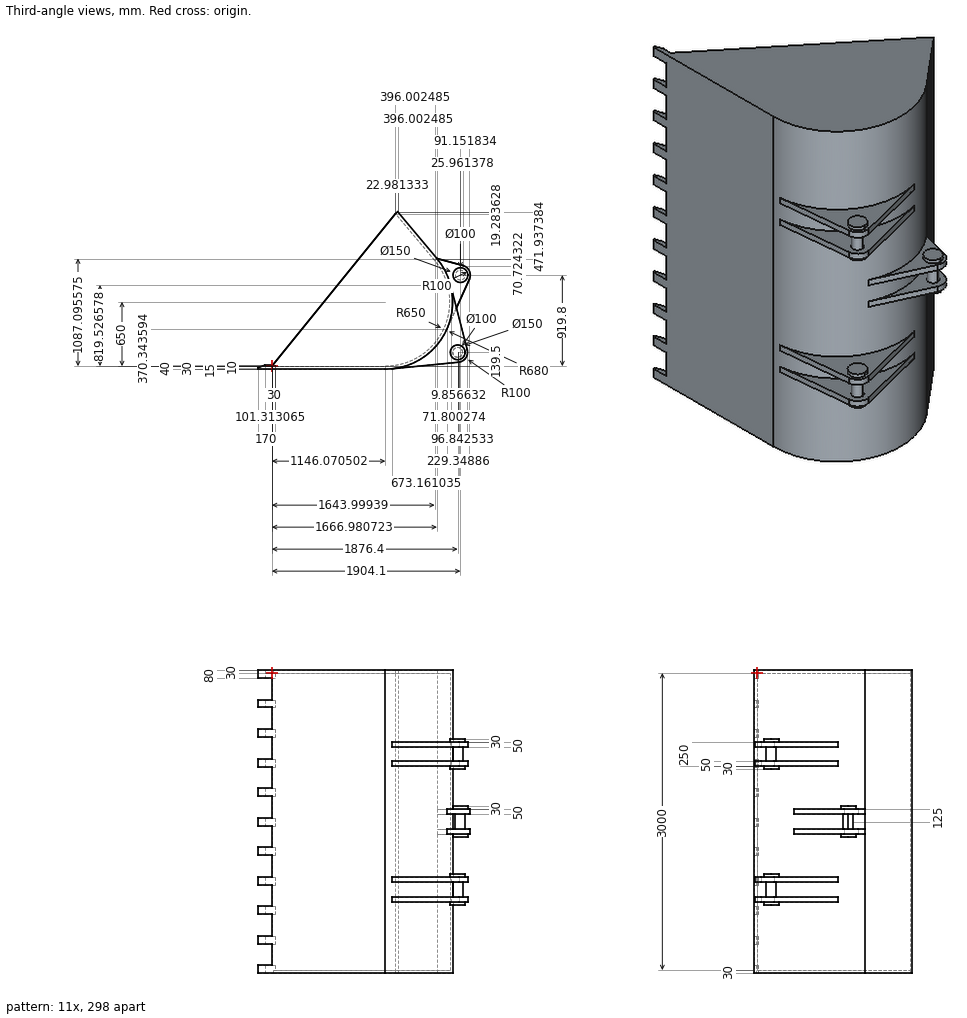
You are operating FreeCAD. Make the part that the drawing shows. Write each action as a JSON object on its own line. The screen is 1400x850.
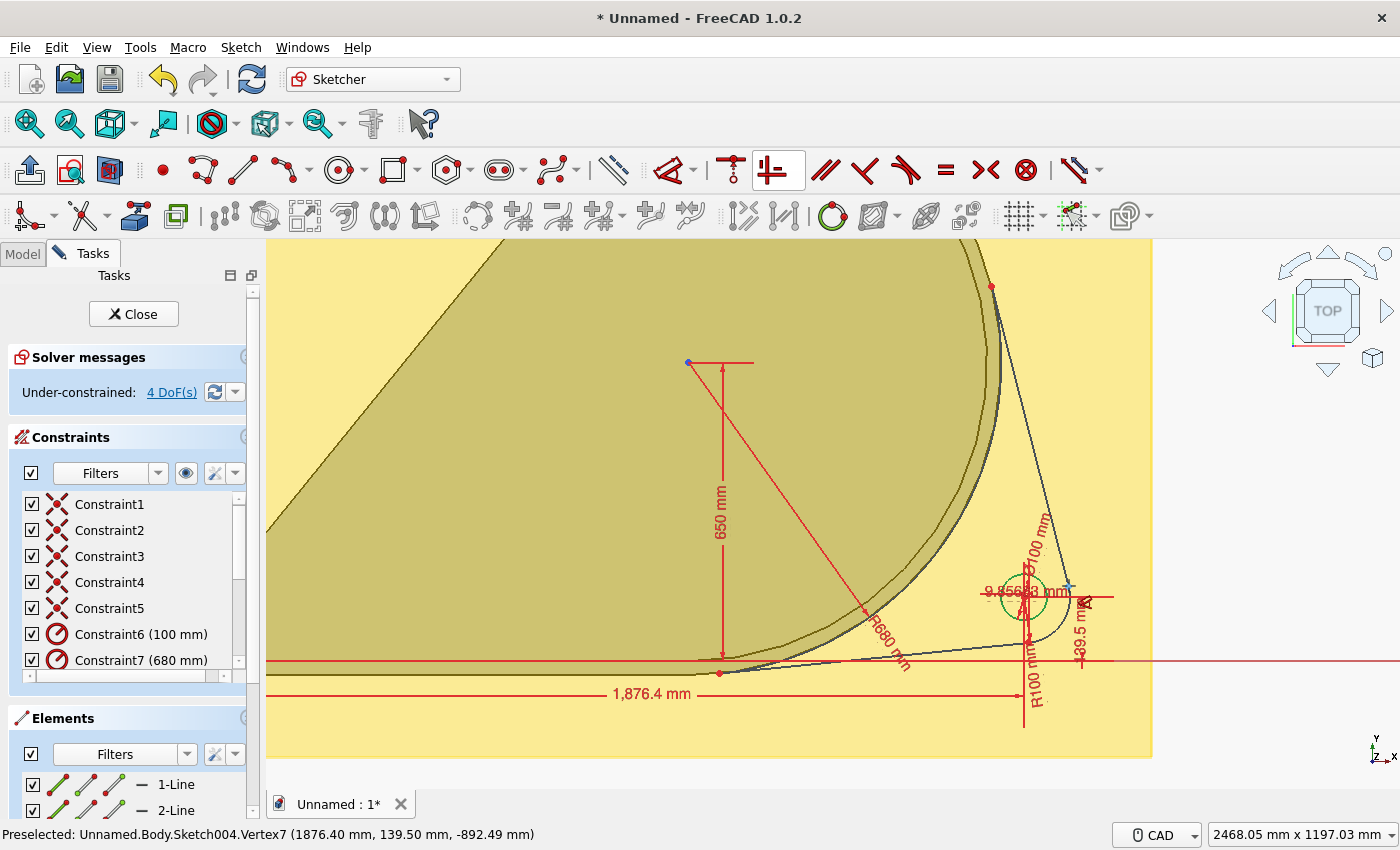
{"action": "left_click", "coordinate": [1069, 586]}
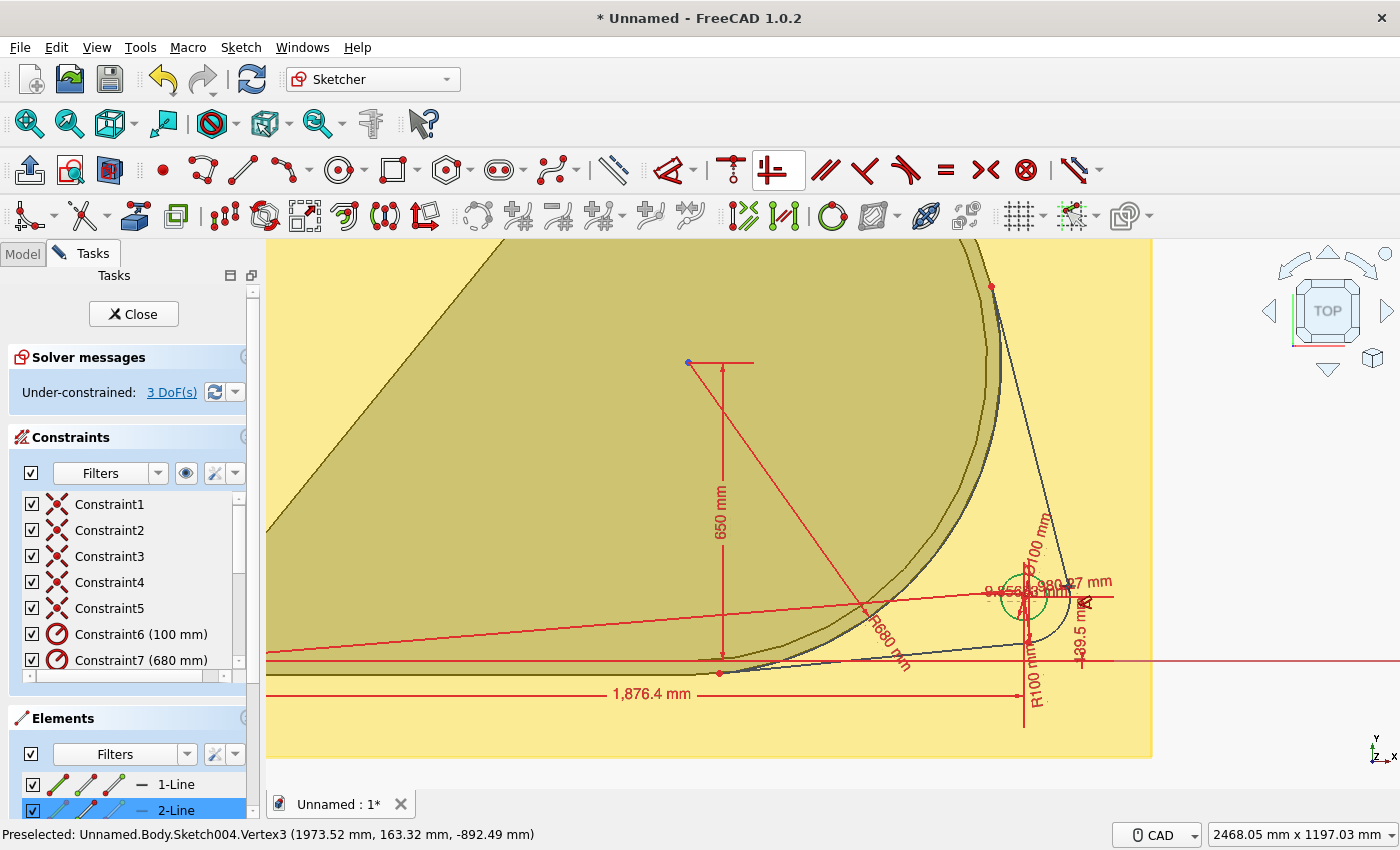
{"action": "left_click", "coordinate": [1024, 597]}
{"action": "left_click", "coordinate": [1031, 504]}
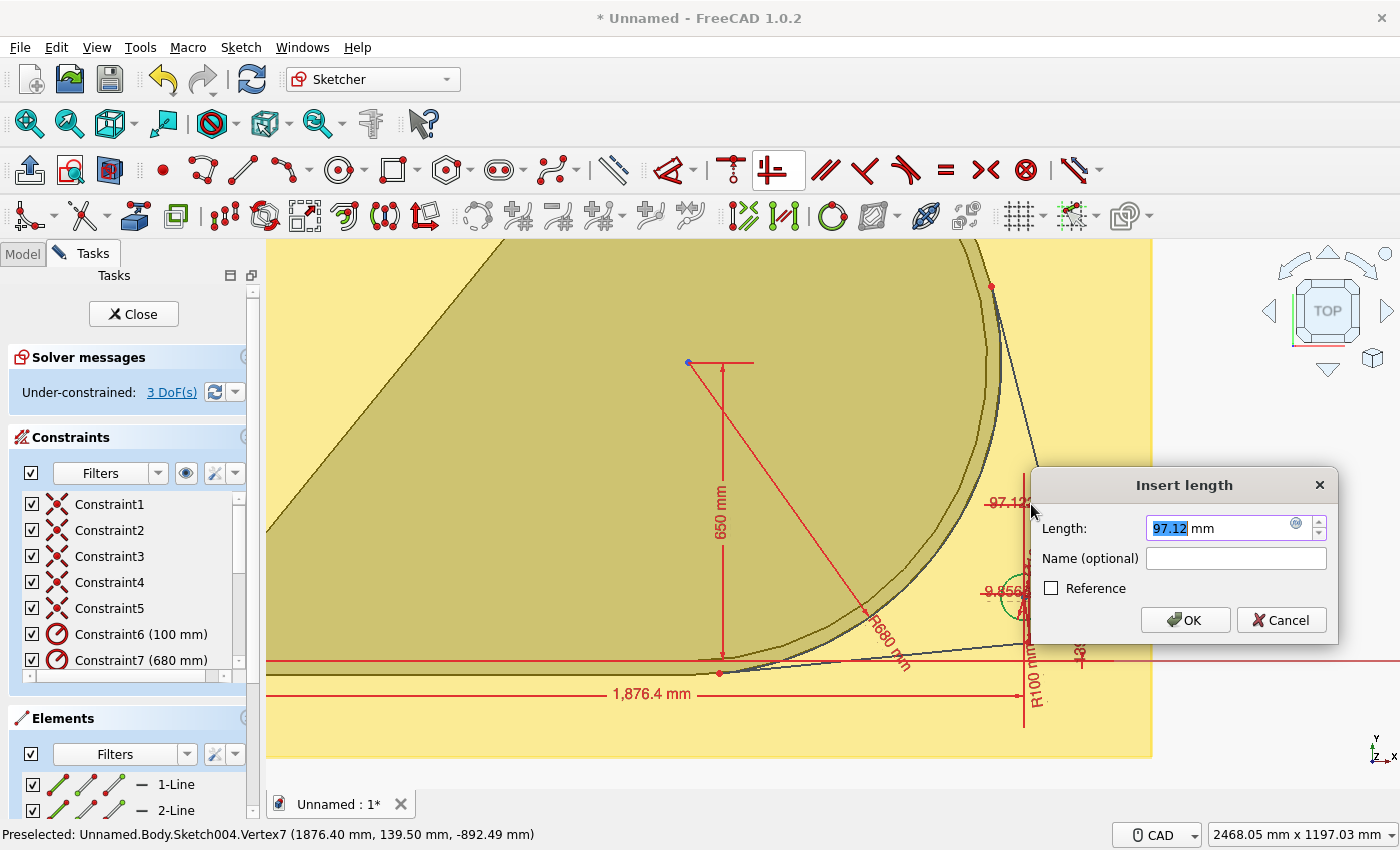
{"action": "type", "text": "96.842533"}
{"action": "key", "text": "Return"}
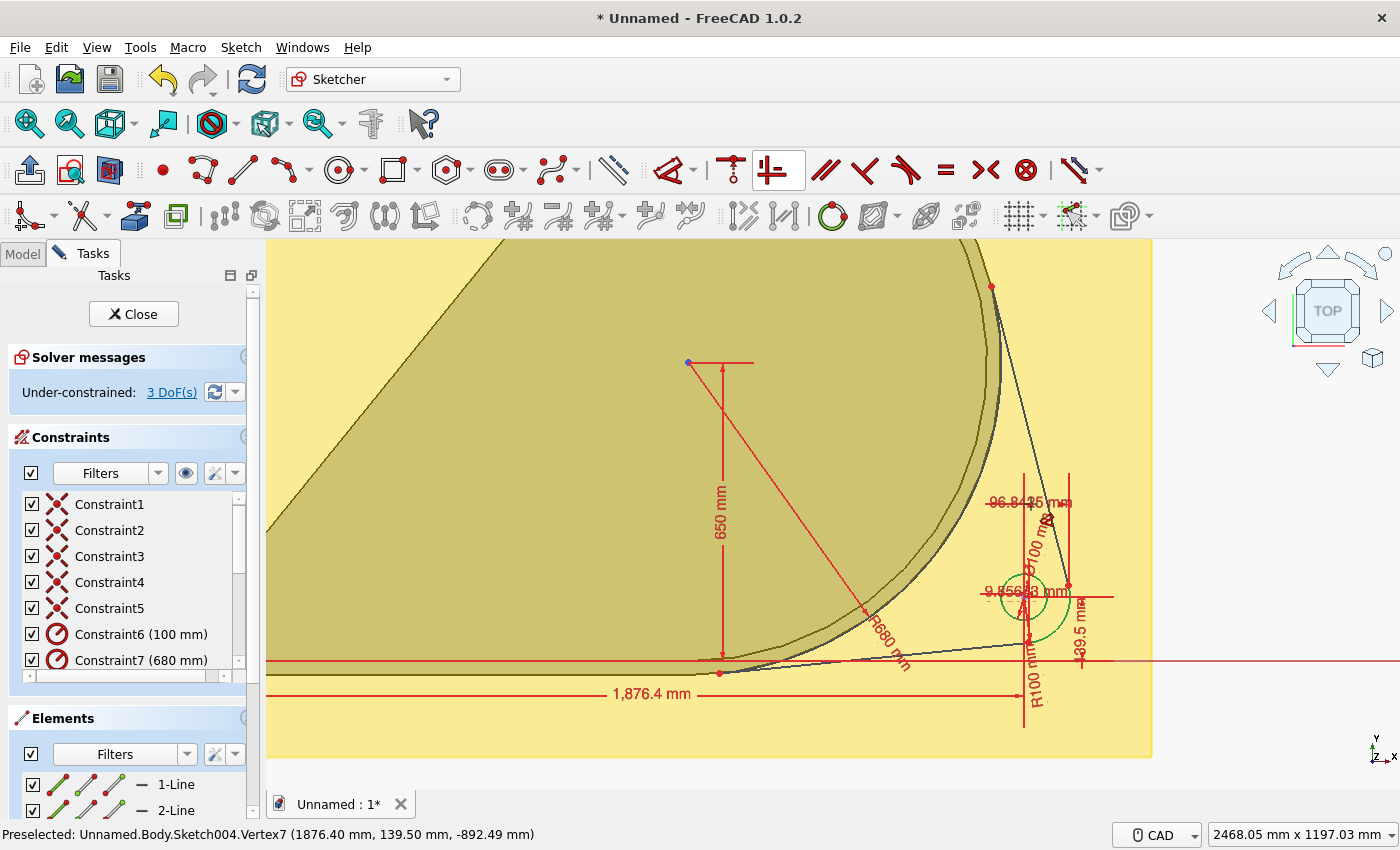
{"action": "left_click", "coordinate": [992, 286]}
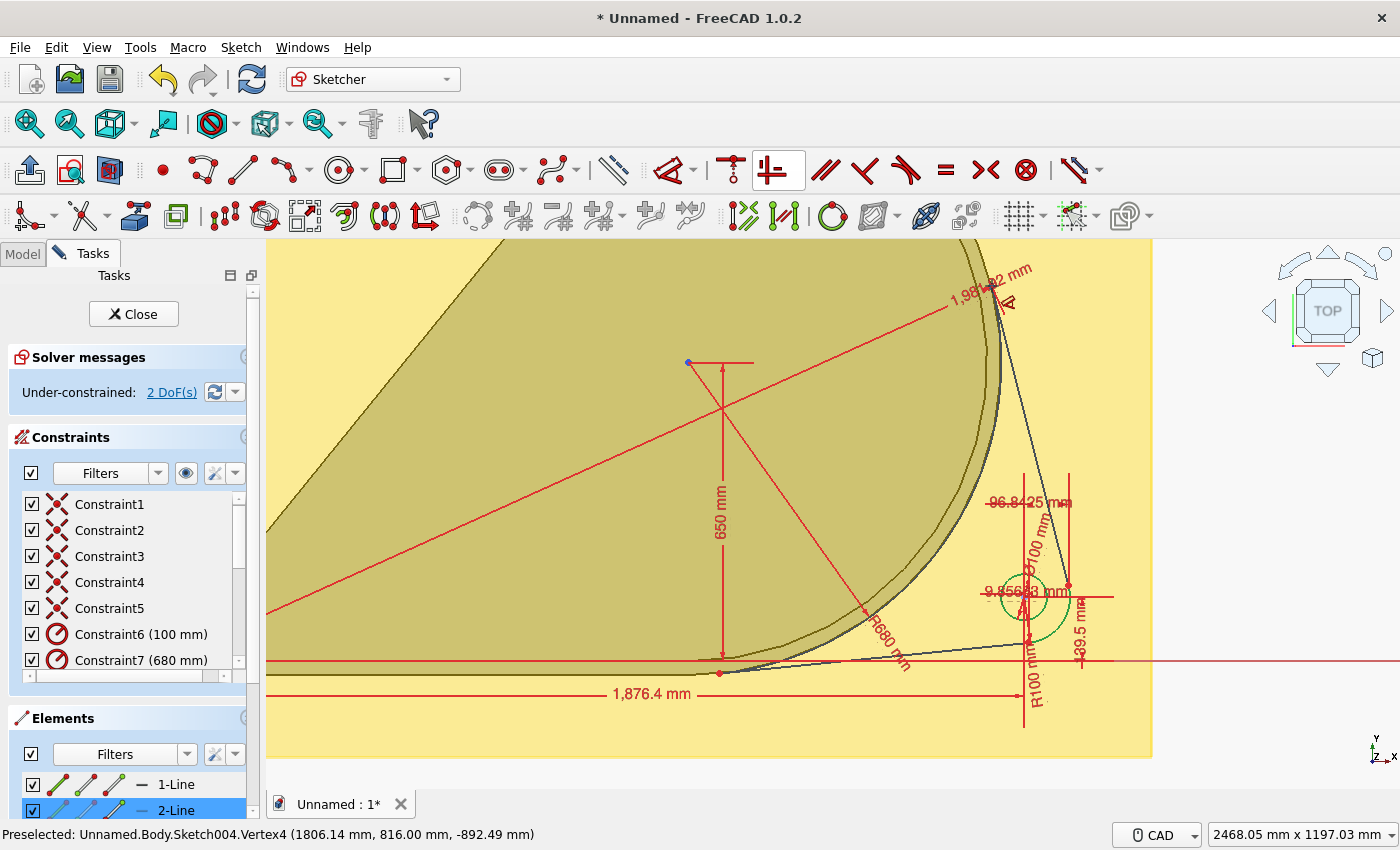
{"action": "left_click", "coordinate": [1024, 597]}
{"action": "left_click", "coordinate": [1008, 631]}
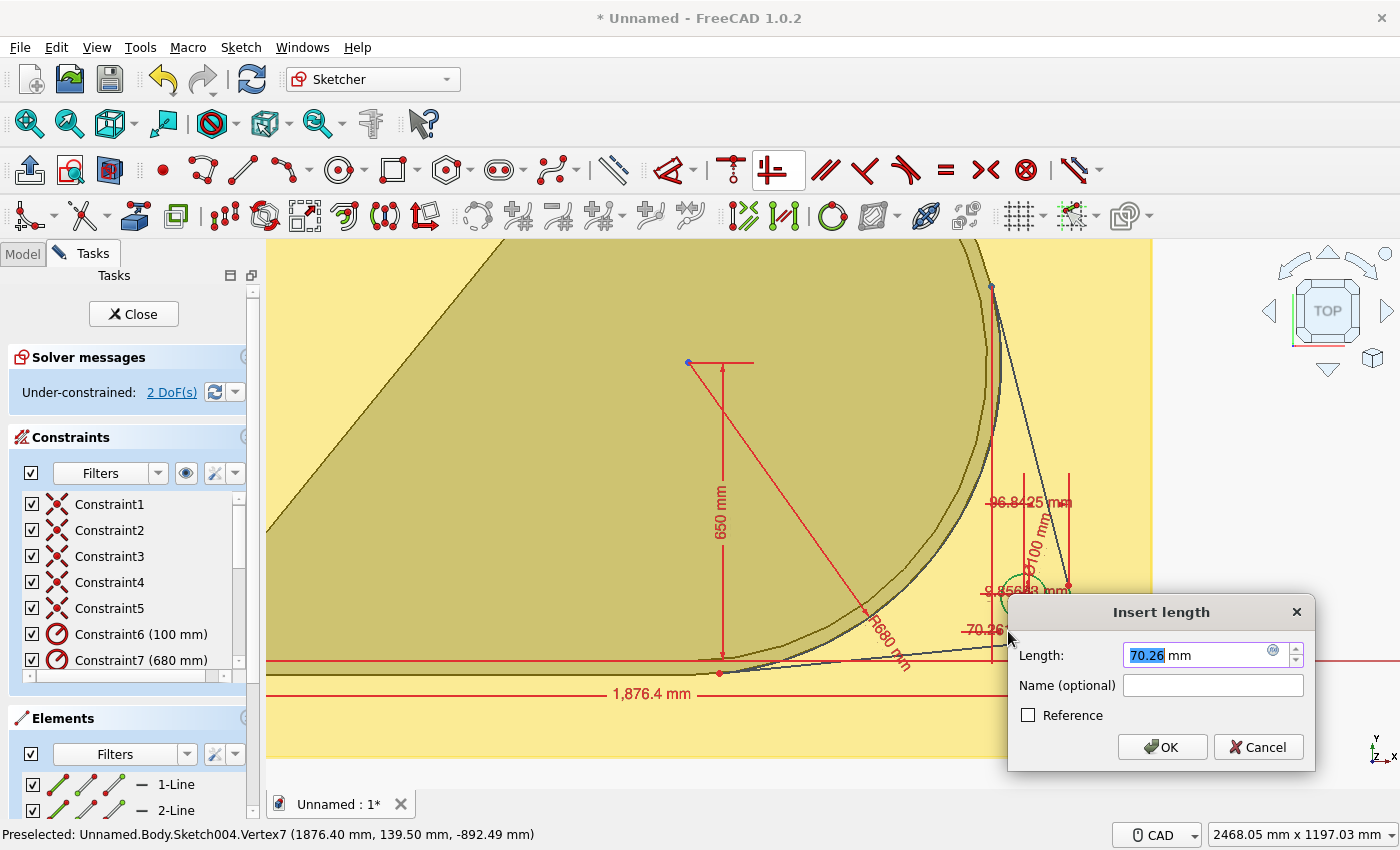
{"action": "type", "text": "71.800274"}
{"action": "key", "text": "Return"}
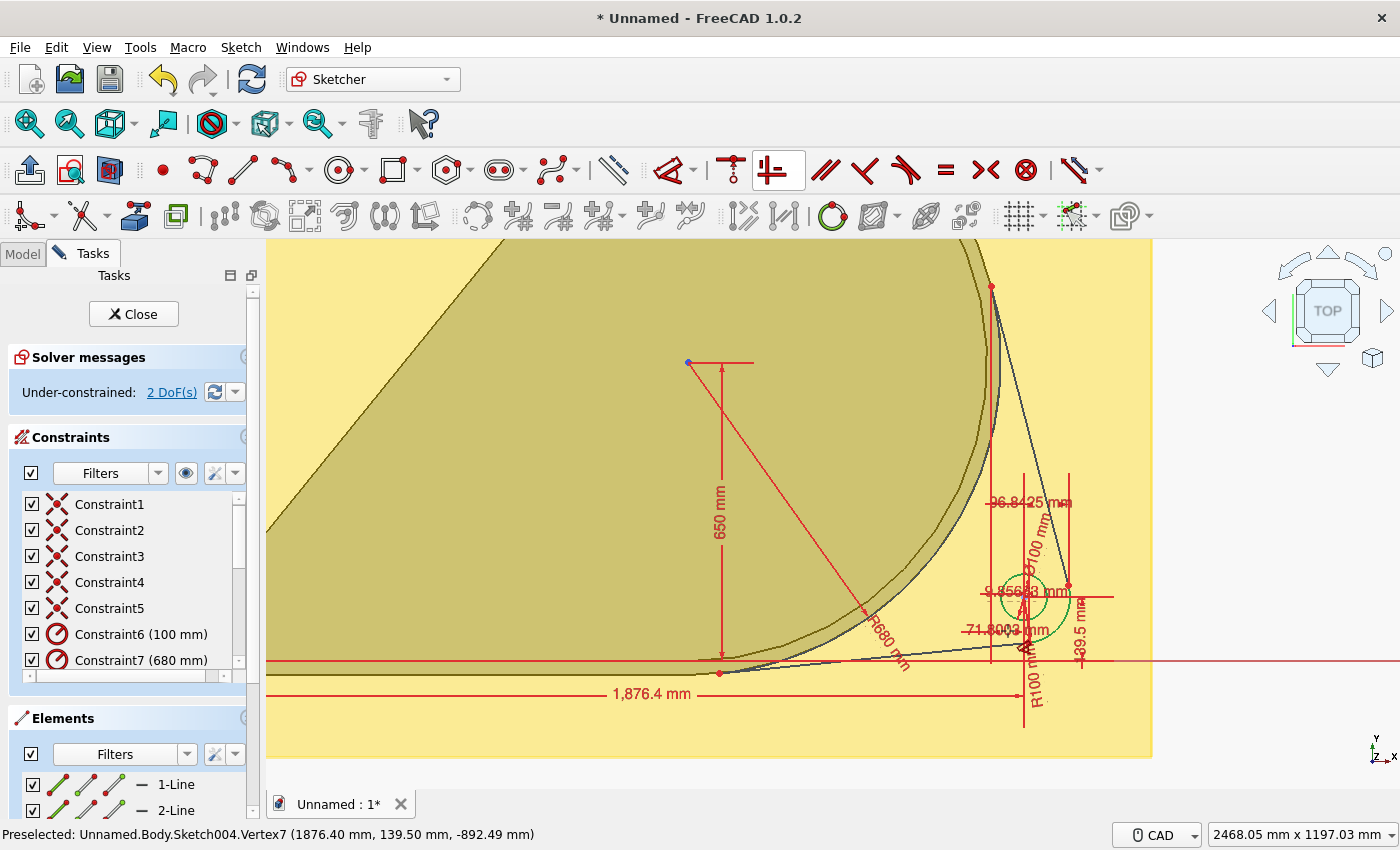
{"action": "left_click", "coordinate": [991, 286]}
{"action": "left_click", "coordinate": [1025, 474]}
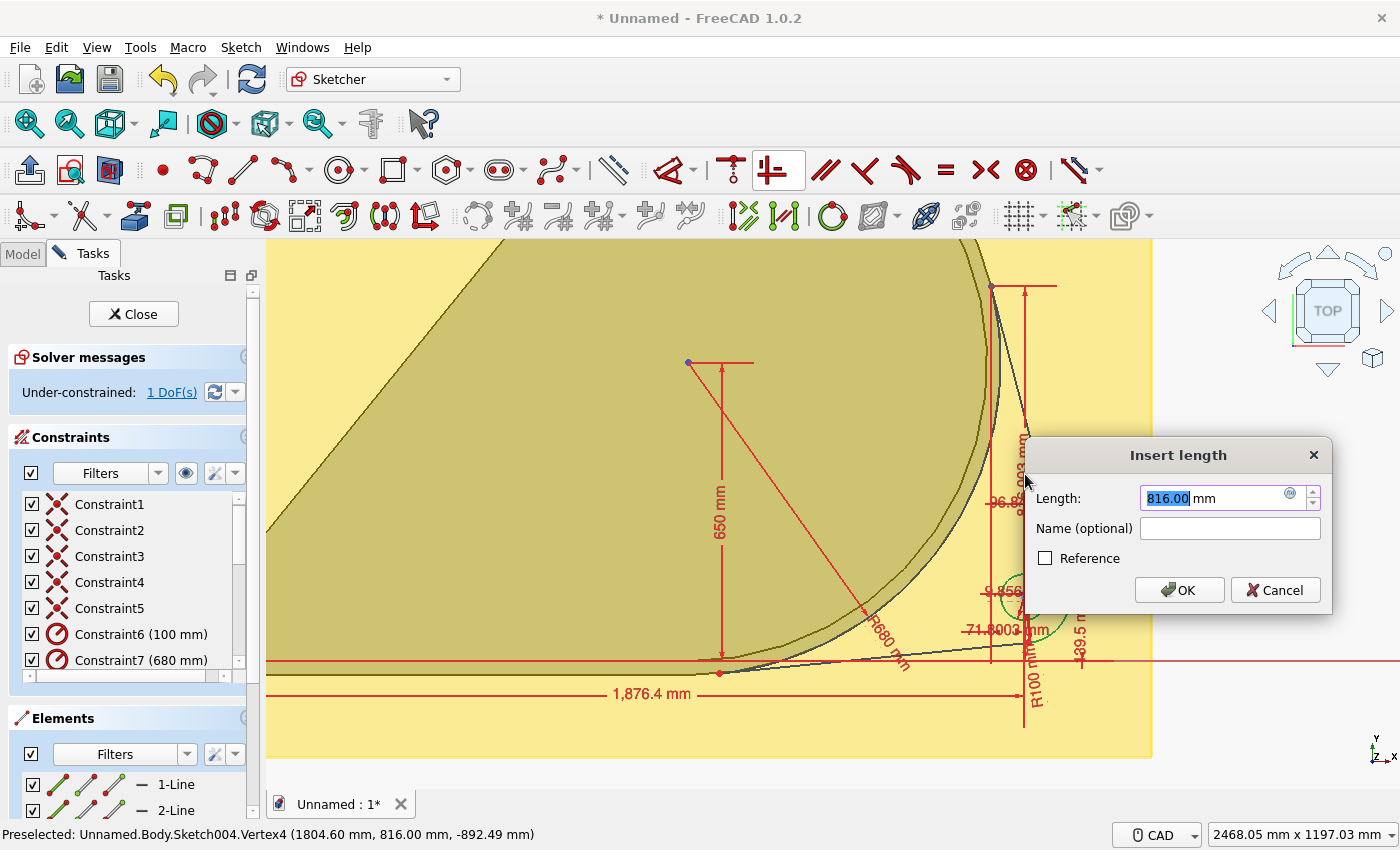
{"action": "type", "text": "819.526578"}
{"action": "key", "text": "Return"}